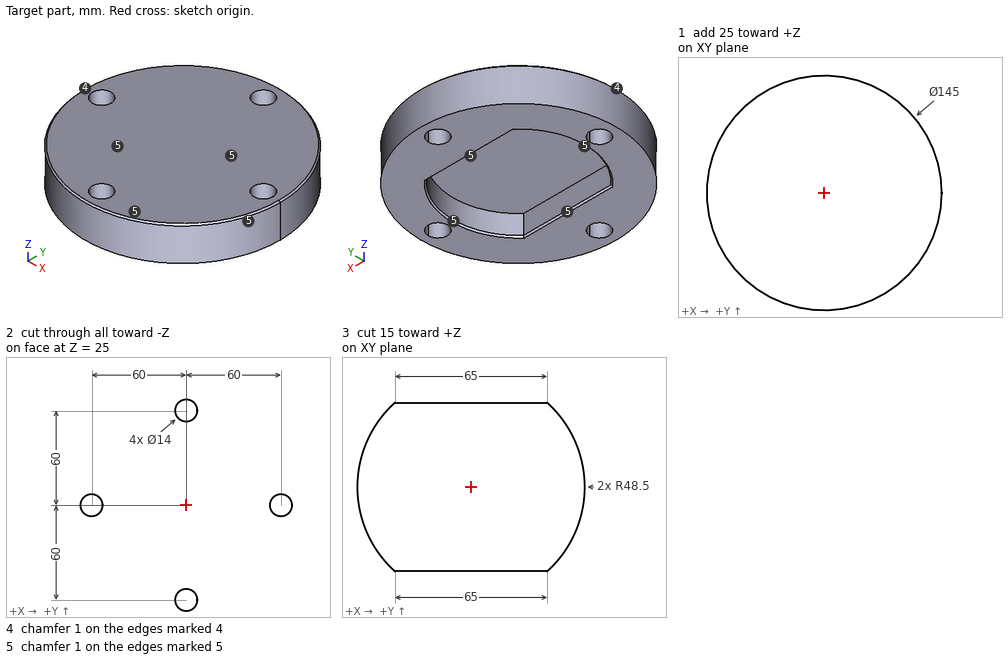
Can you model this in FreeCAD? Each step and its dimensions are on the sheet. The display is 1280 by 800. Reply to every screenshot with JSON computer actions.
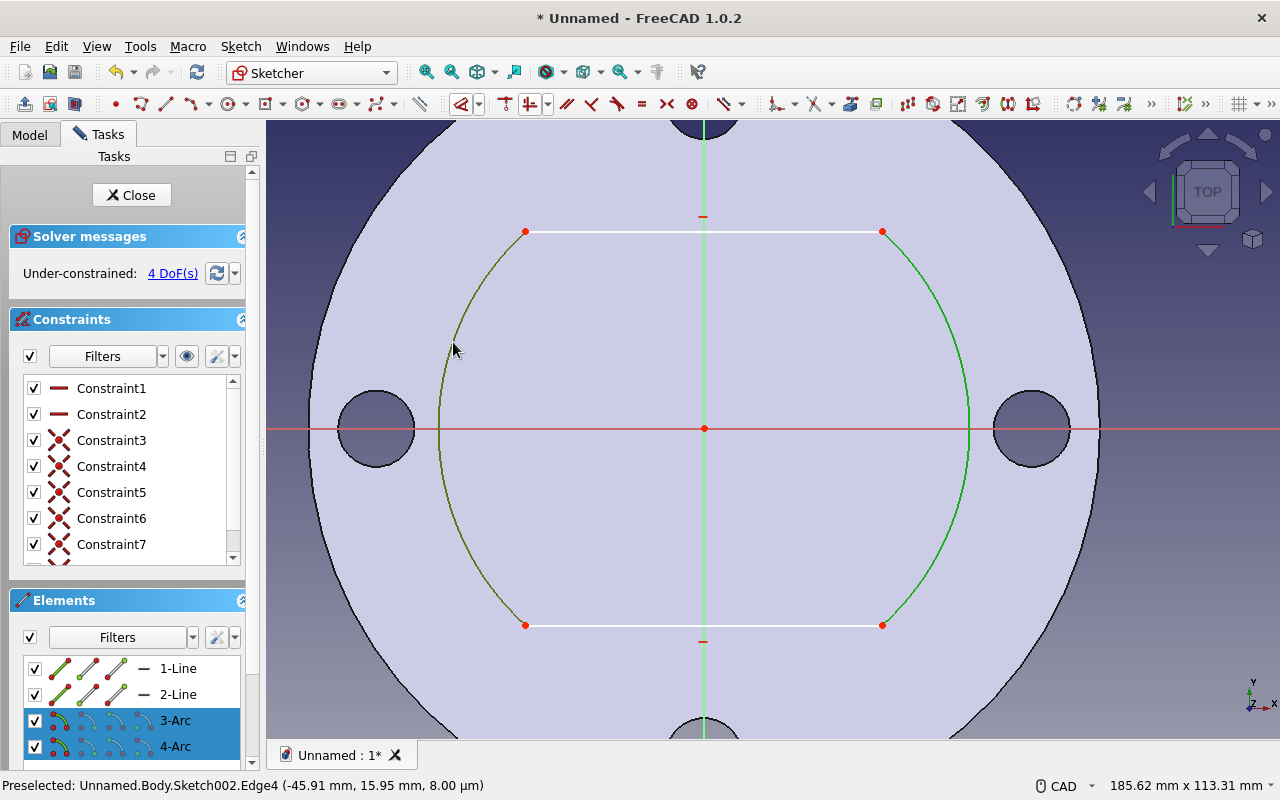
{"action": "left_click", "coordinate": [642, 104]}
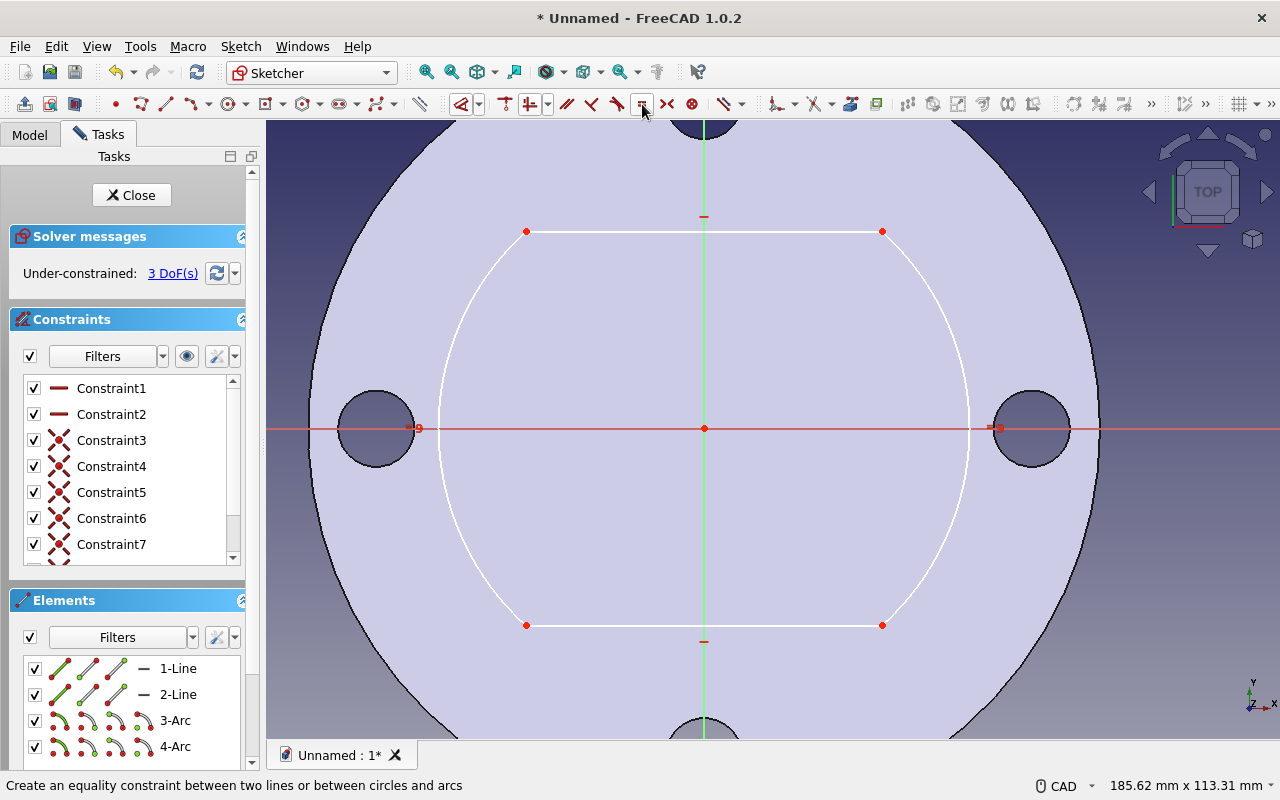
{"action": "left_click", "coordinate": [955, 516]}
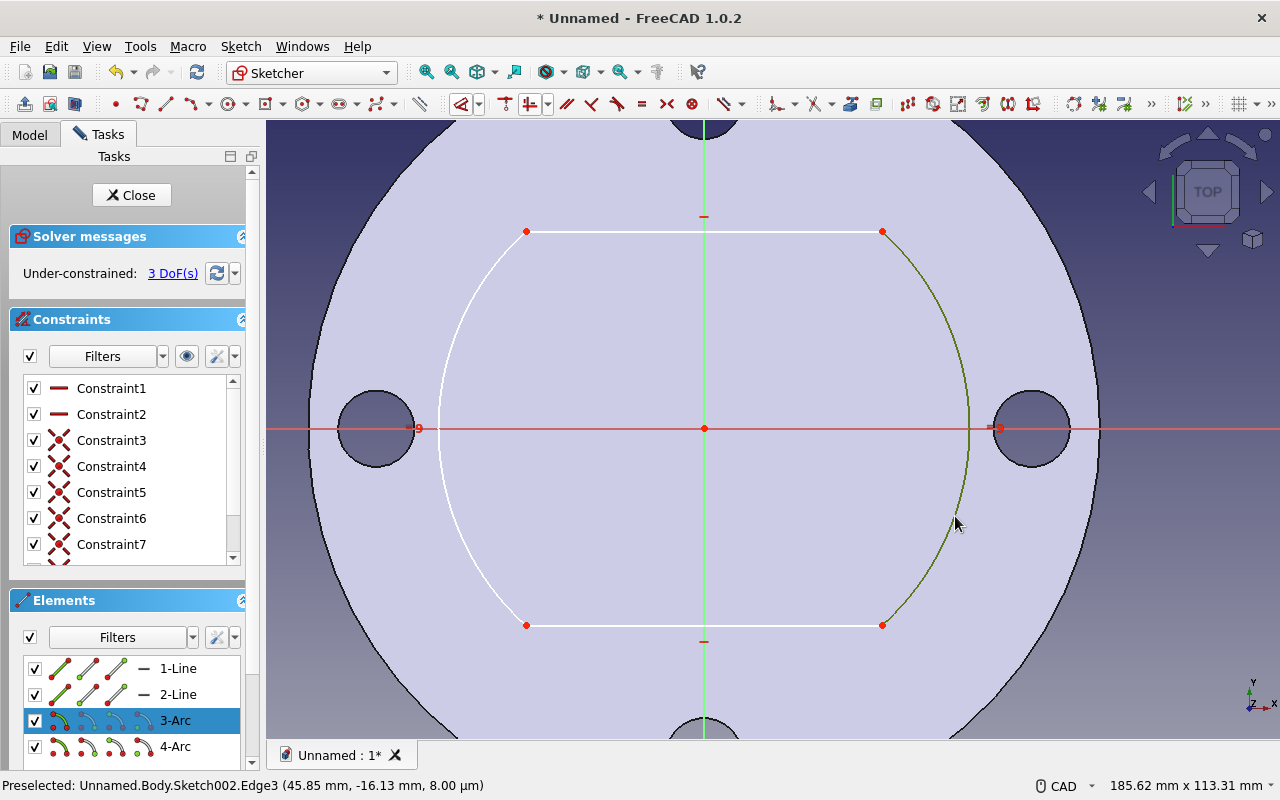
{"action": "left_click", "coordinate": [478, 104]}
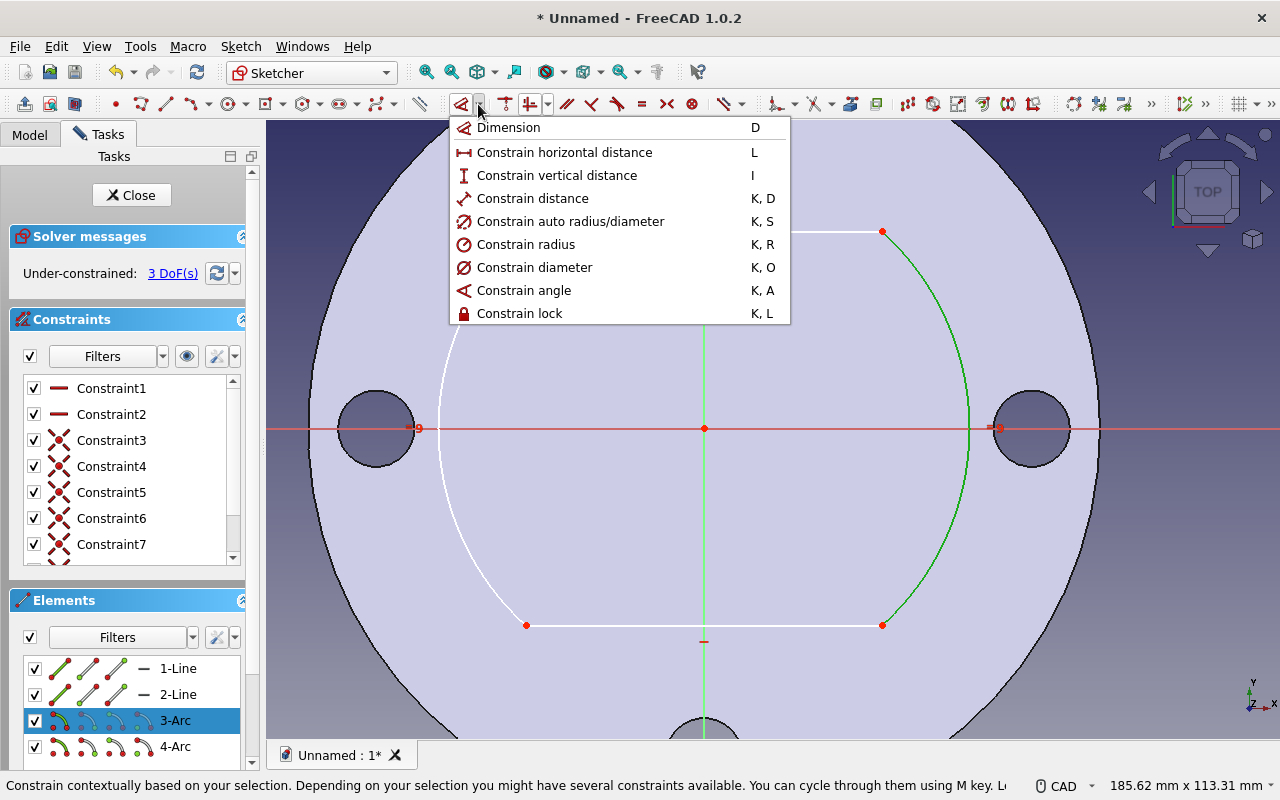
{"action": "left_click", "coordinate": [620, 244]}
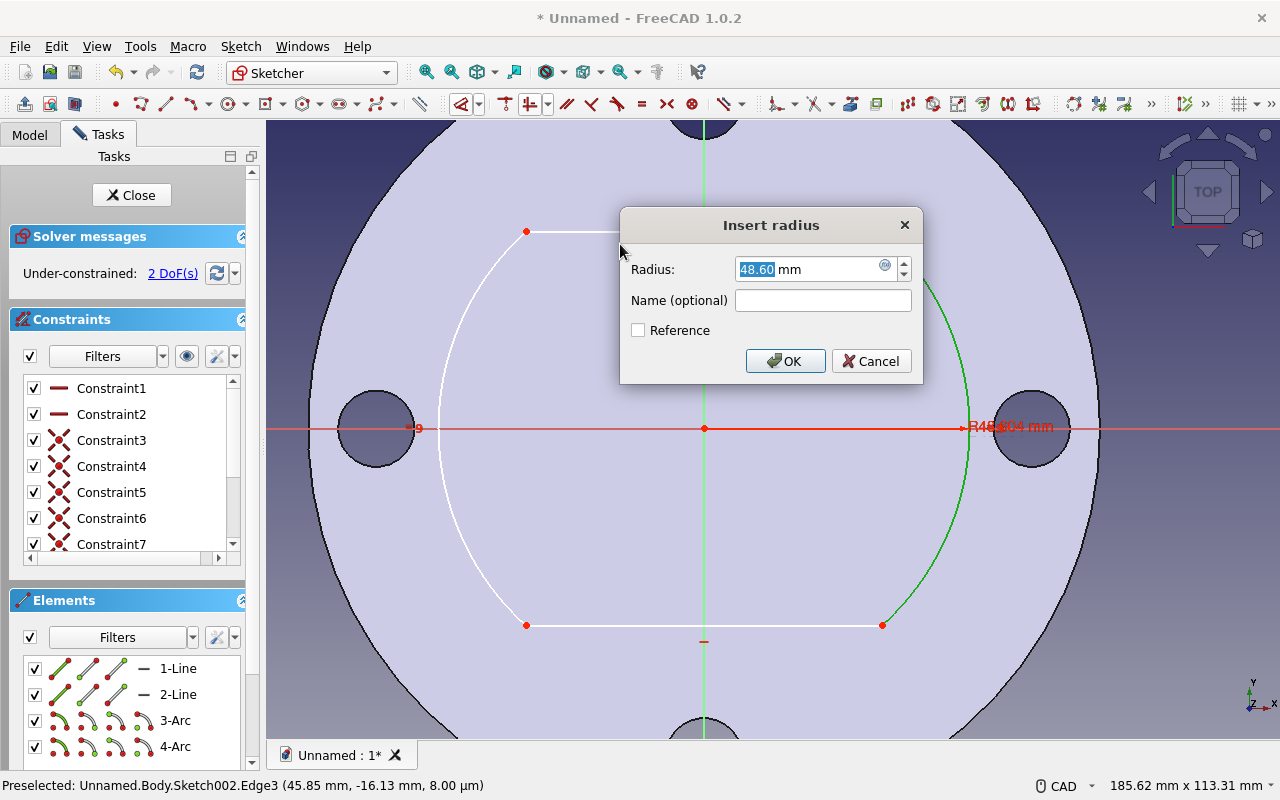
{"action": "type", "text": "48.5"}
{"action": "key", "text": "Return"}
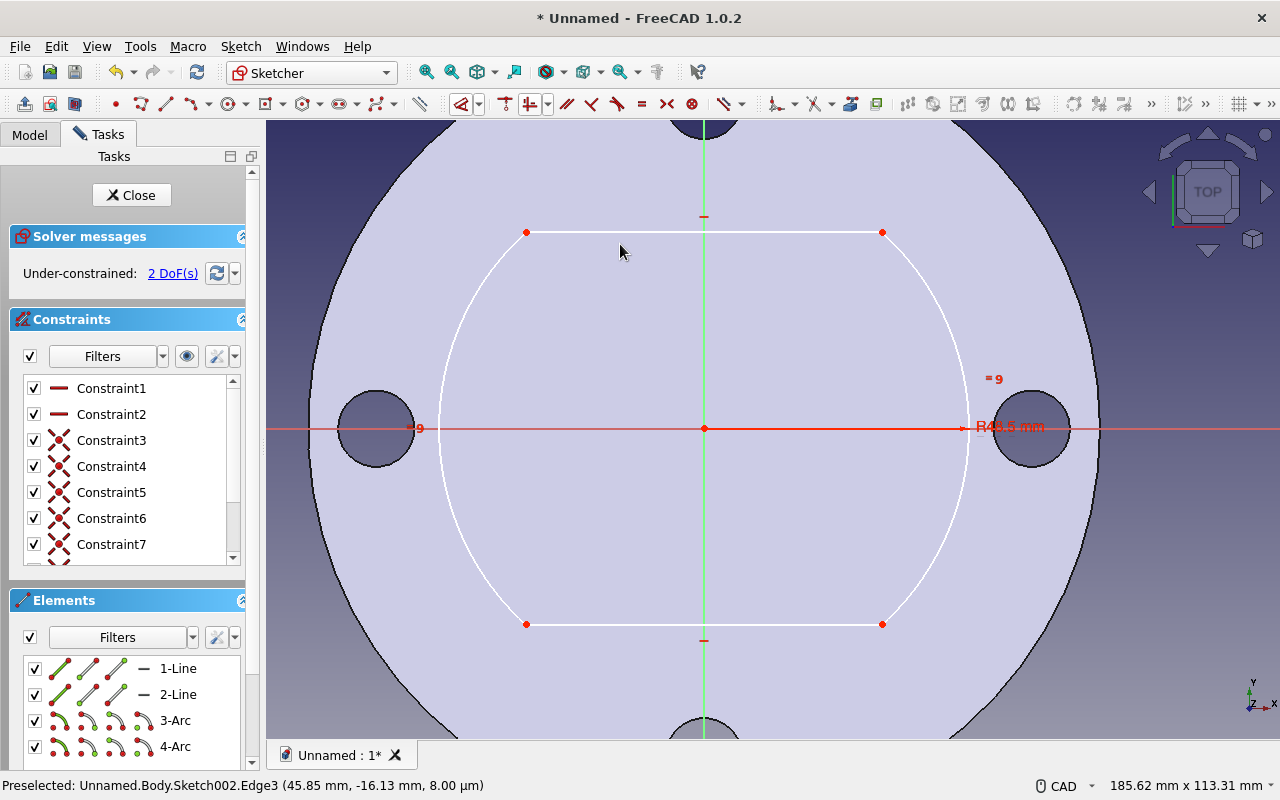
{"action": "left_click", "coordinate": [633, 232]}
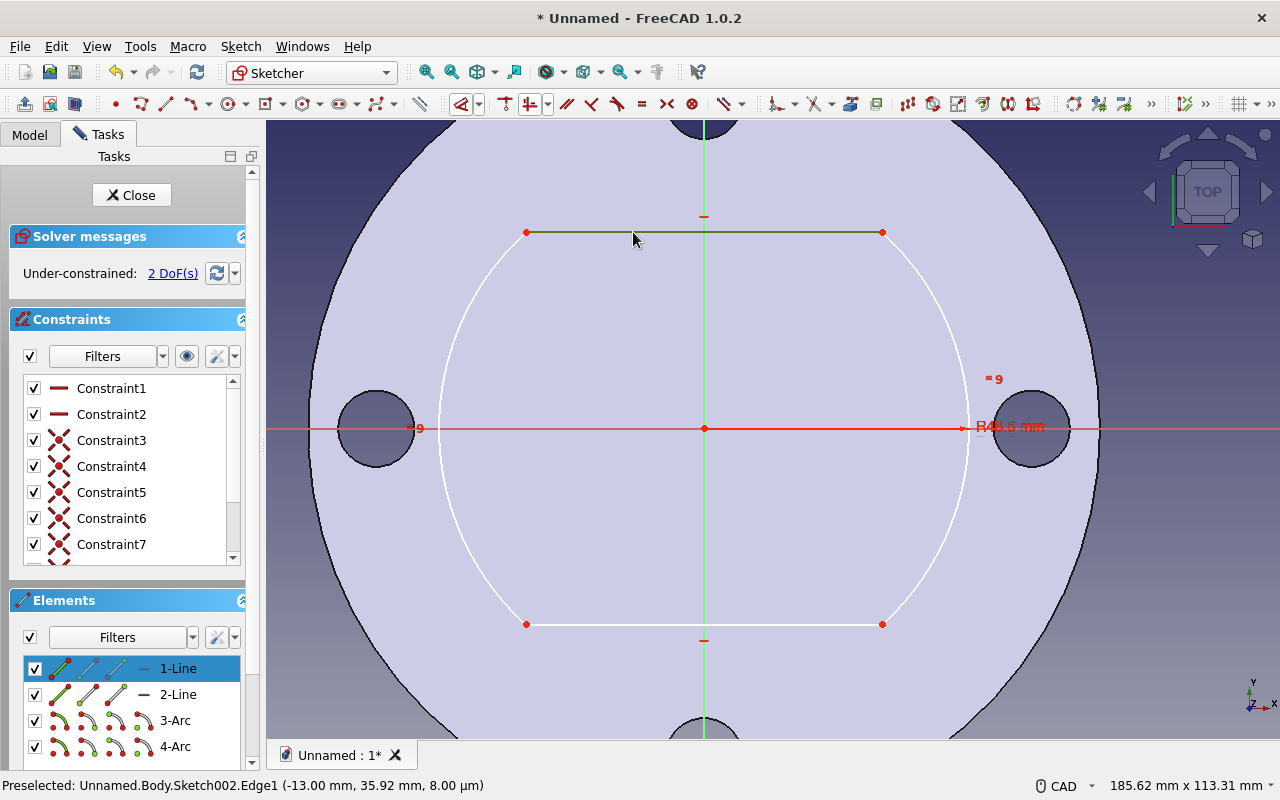
{"action": "left_click", "coordinate": [478, 104]}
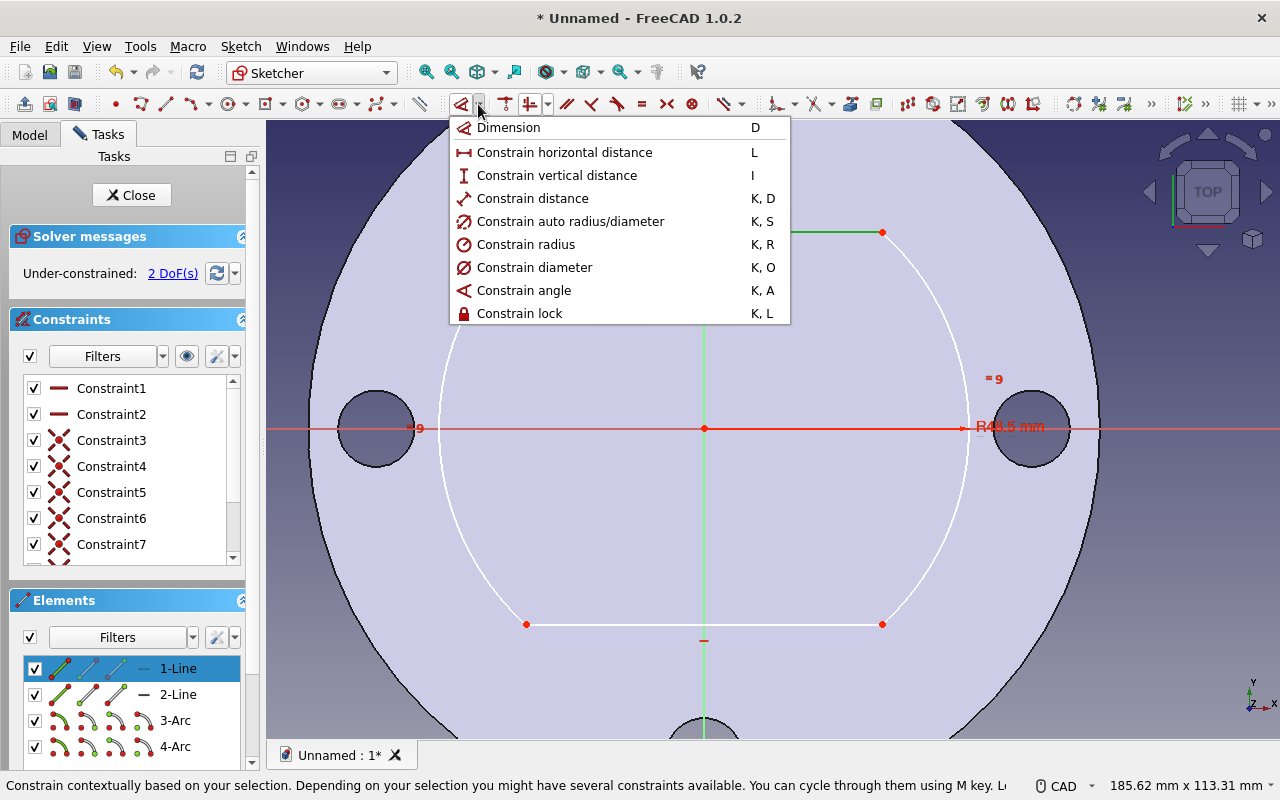
{"action": "left_click", "coordinate": [620, 152]}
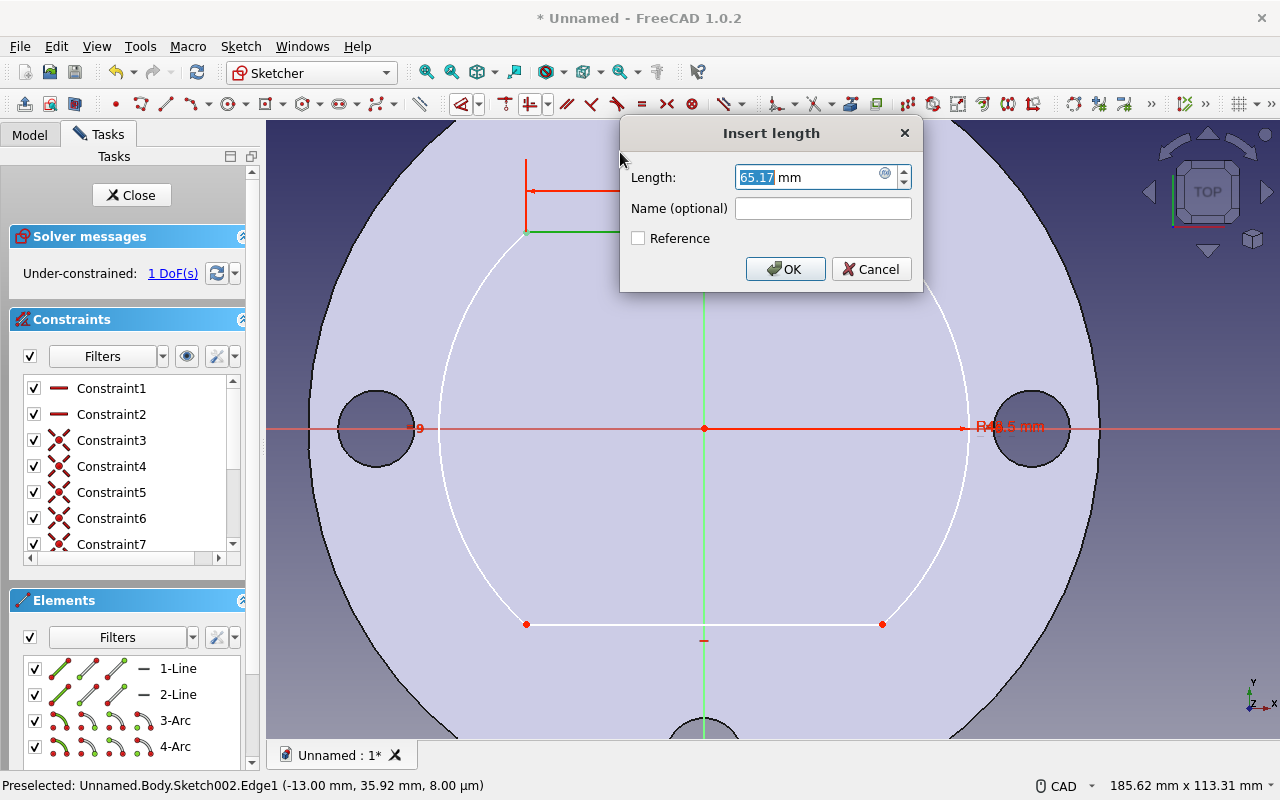
{"action": "type", "text": "65"}
{"action": "key", "text": "Return"}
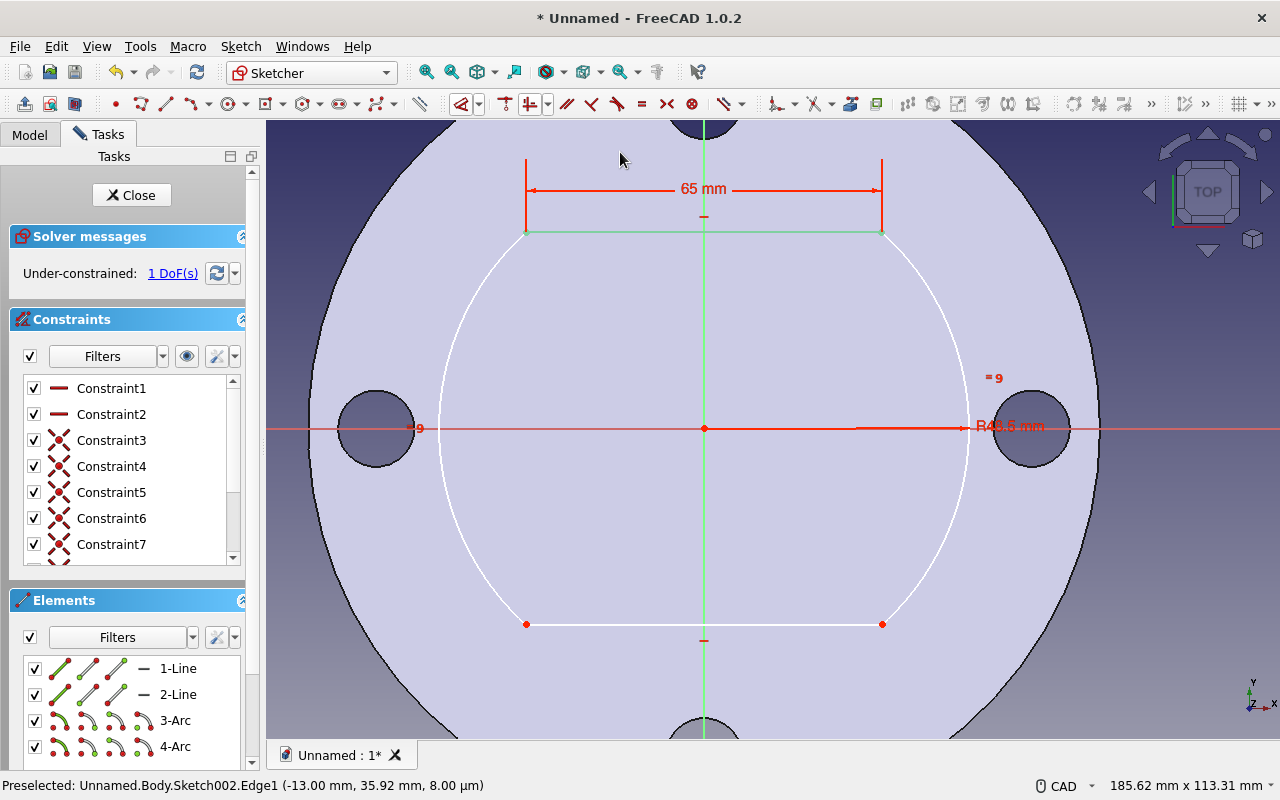
{"action": "left_click", "coordinate": [775, 625]}